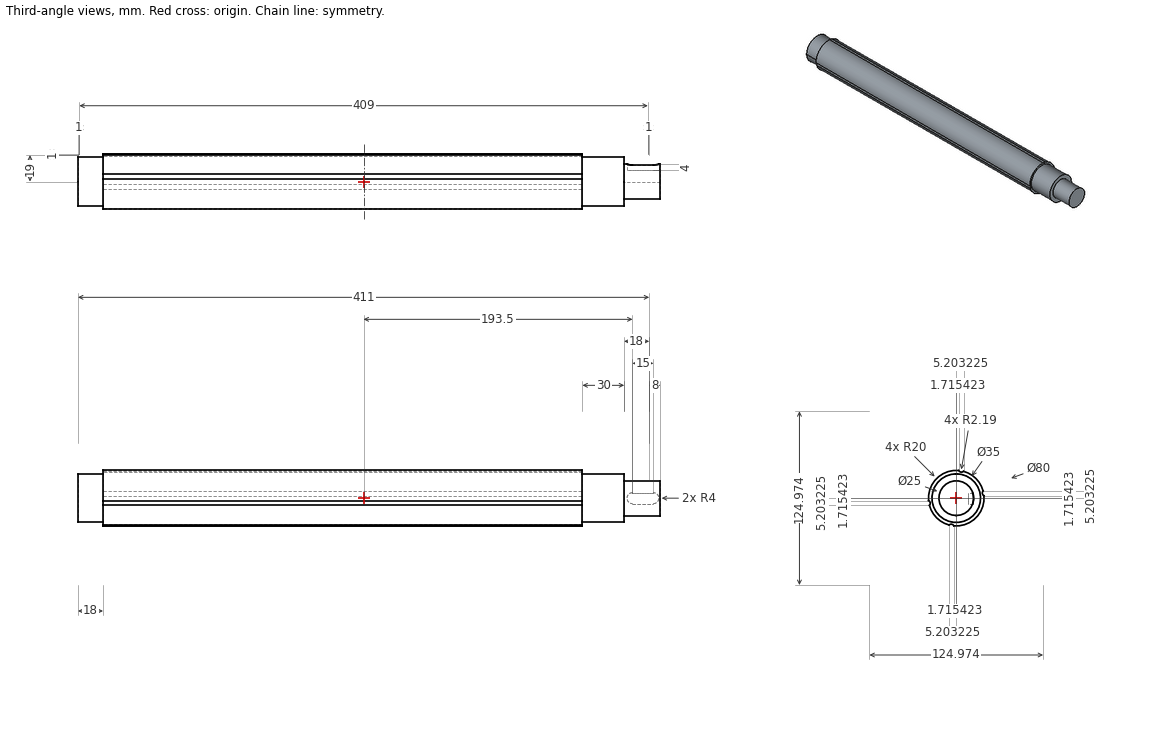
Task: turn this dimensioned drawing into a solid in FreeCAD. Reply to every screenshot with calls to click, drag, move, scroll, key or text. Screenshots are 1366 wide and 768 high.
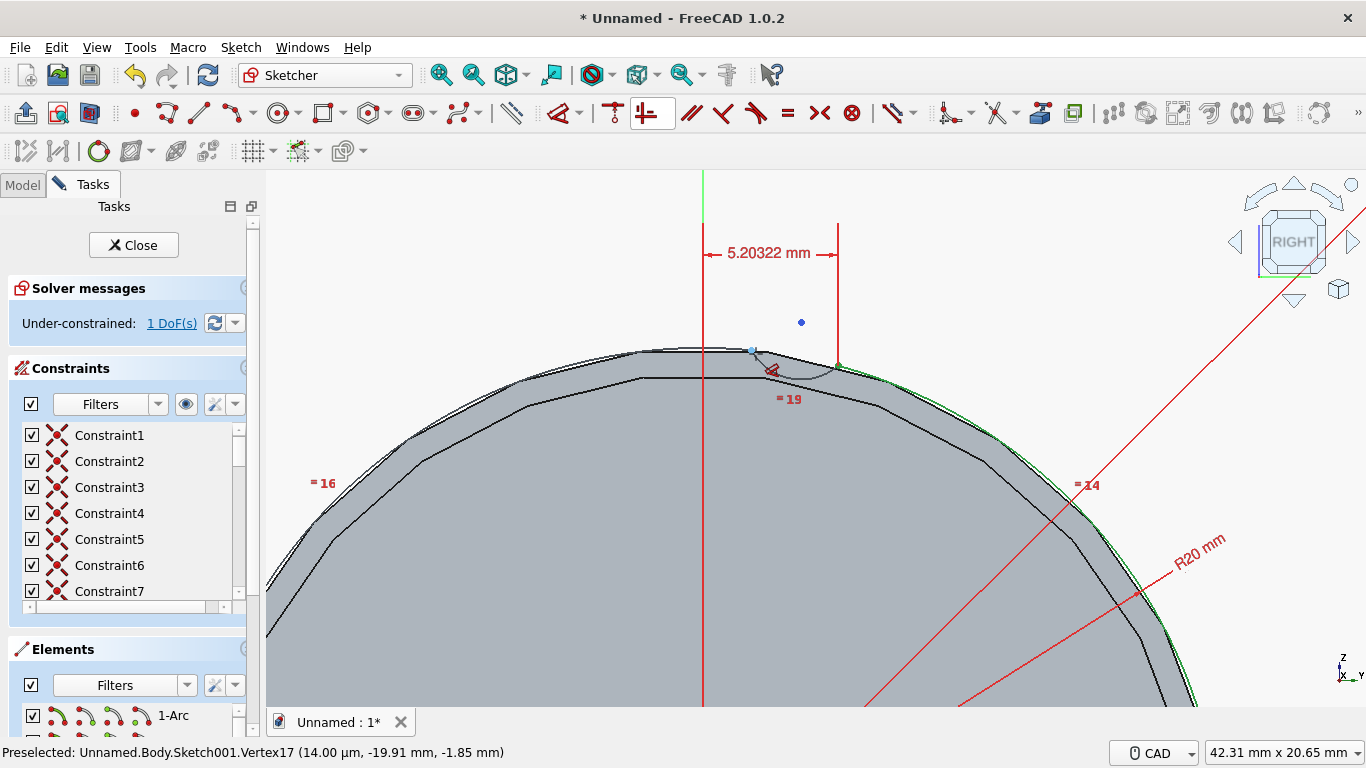
click(751, 350)
click(727, 316)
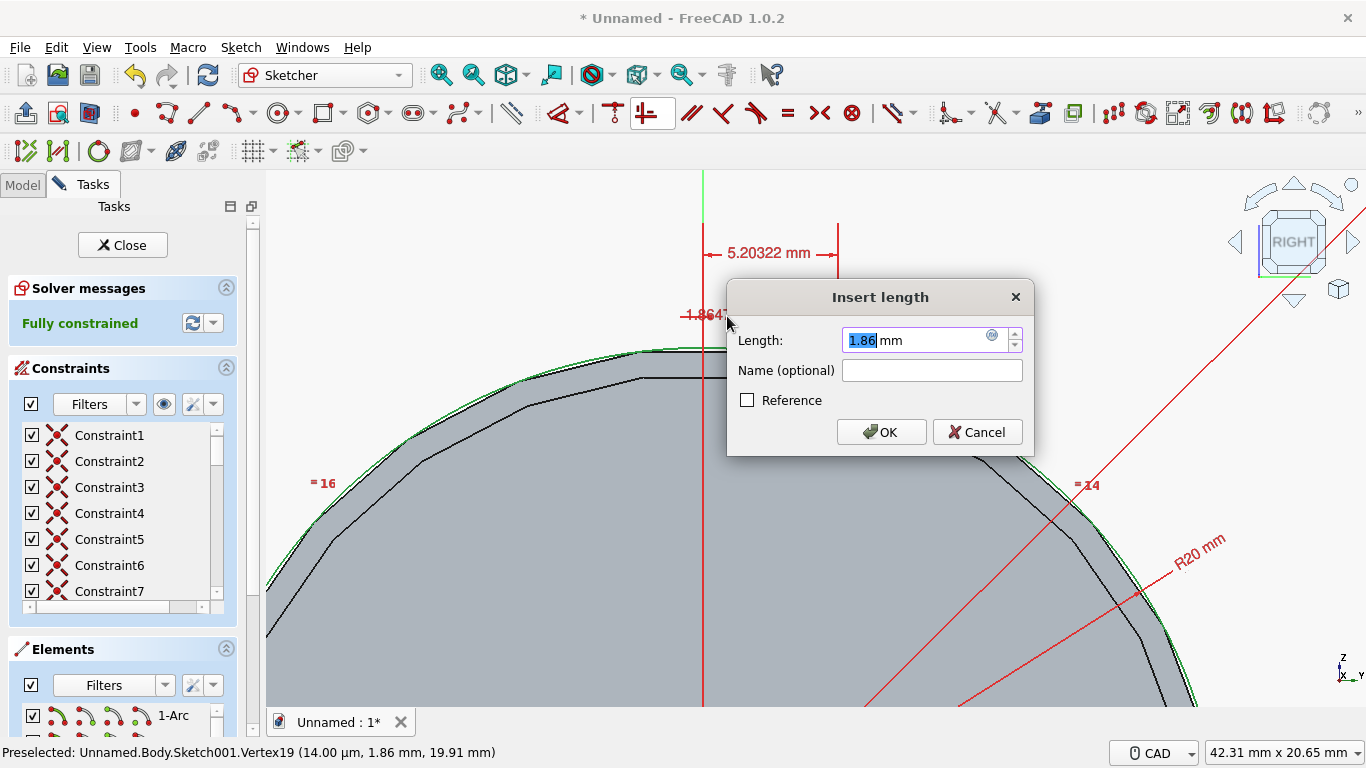
text(1.715423)
key(Return)
key(Escape)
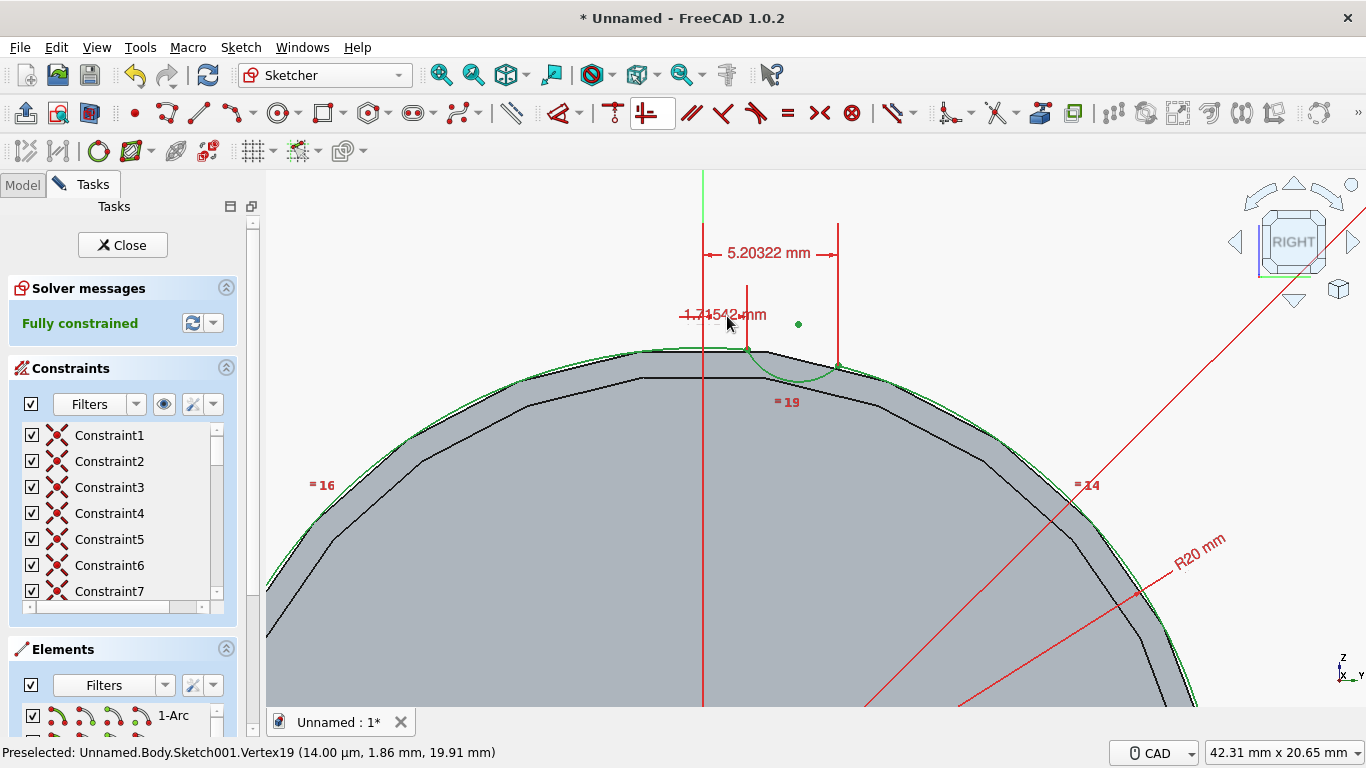
click(123, 245)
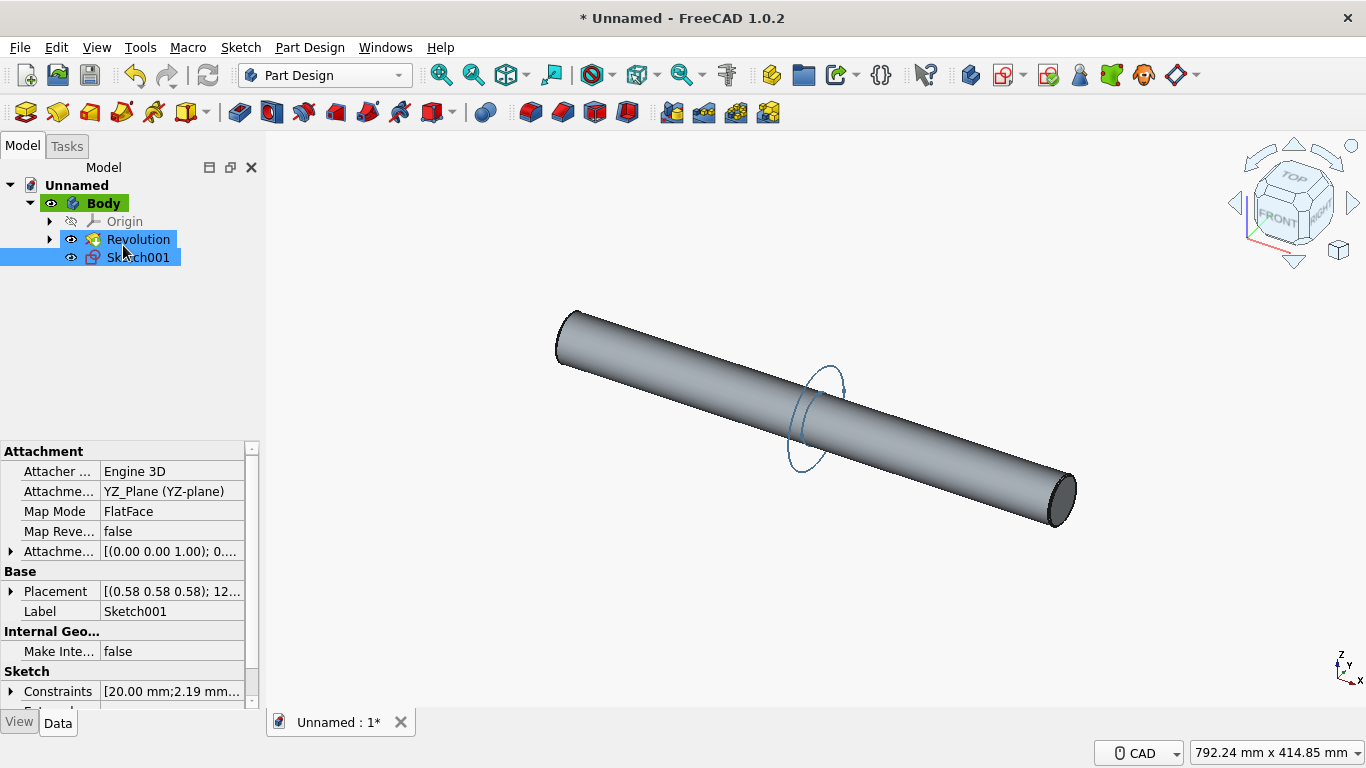
click(240, 112)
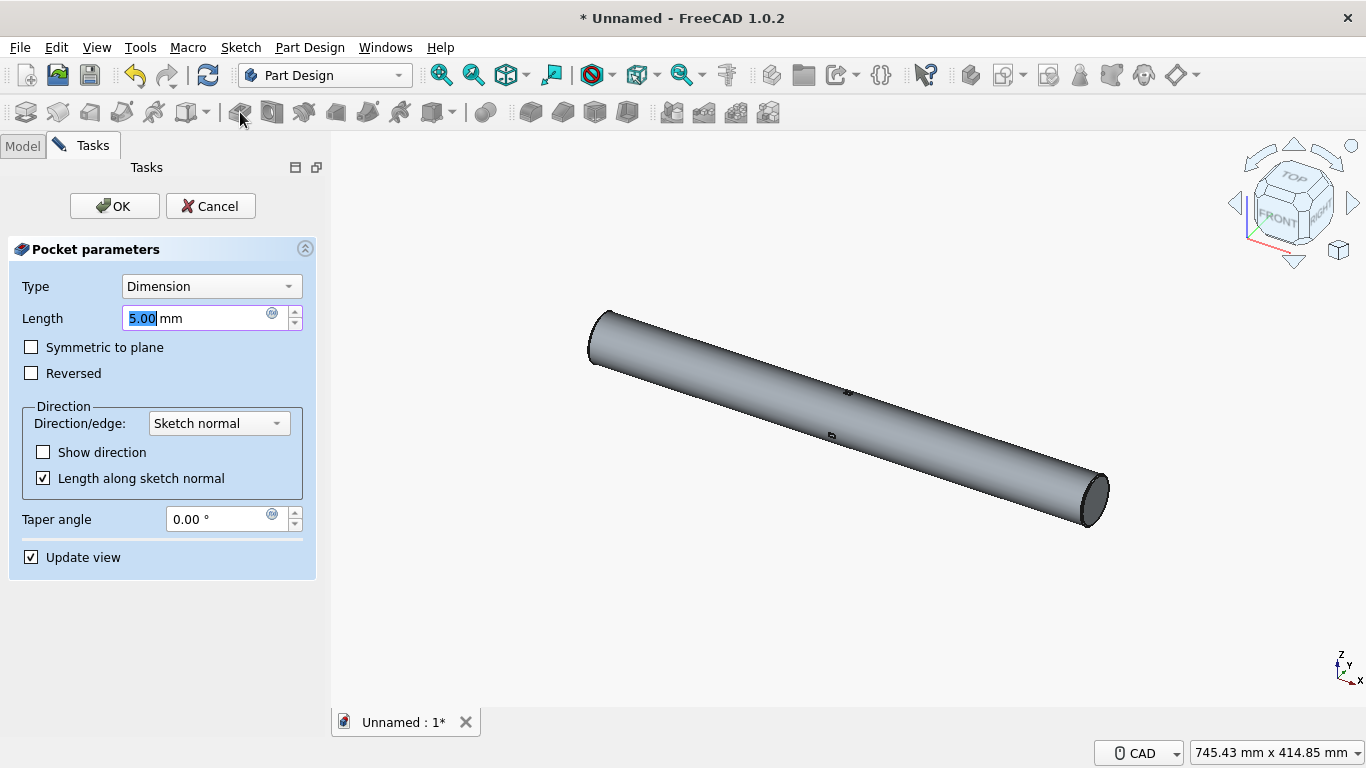
text(411)
key(Tab)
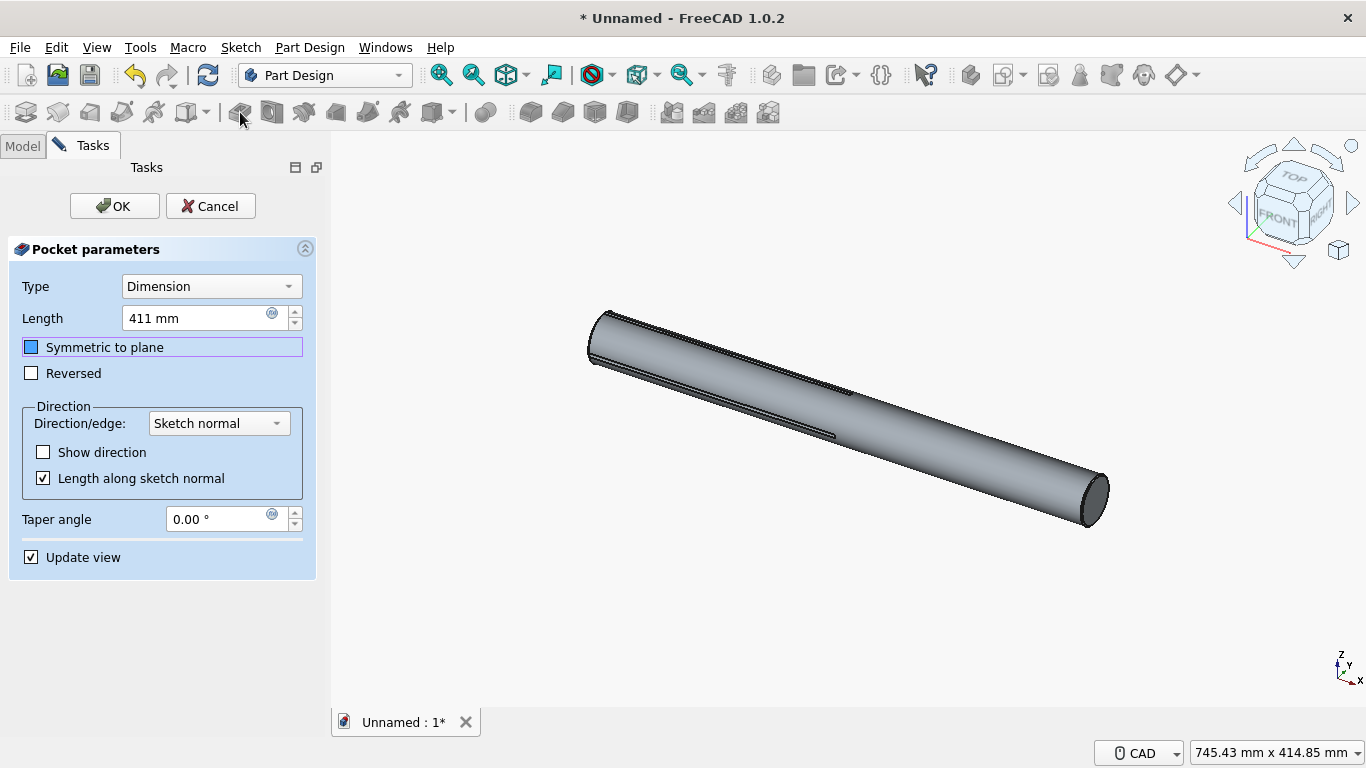
click(30, 347)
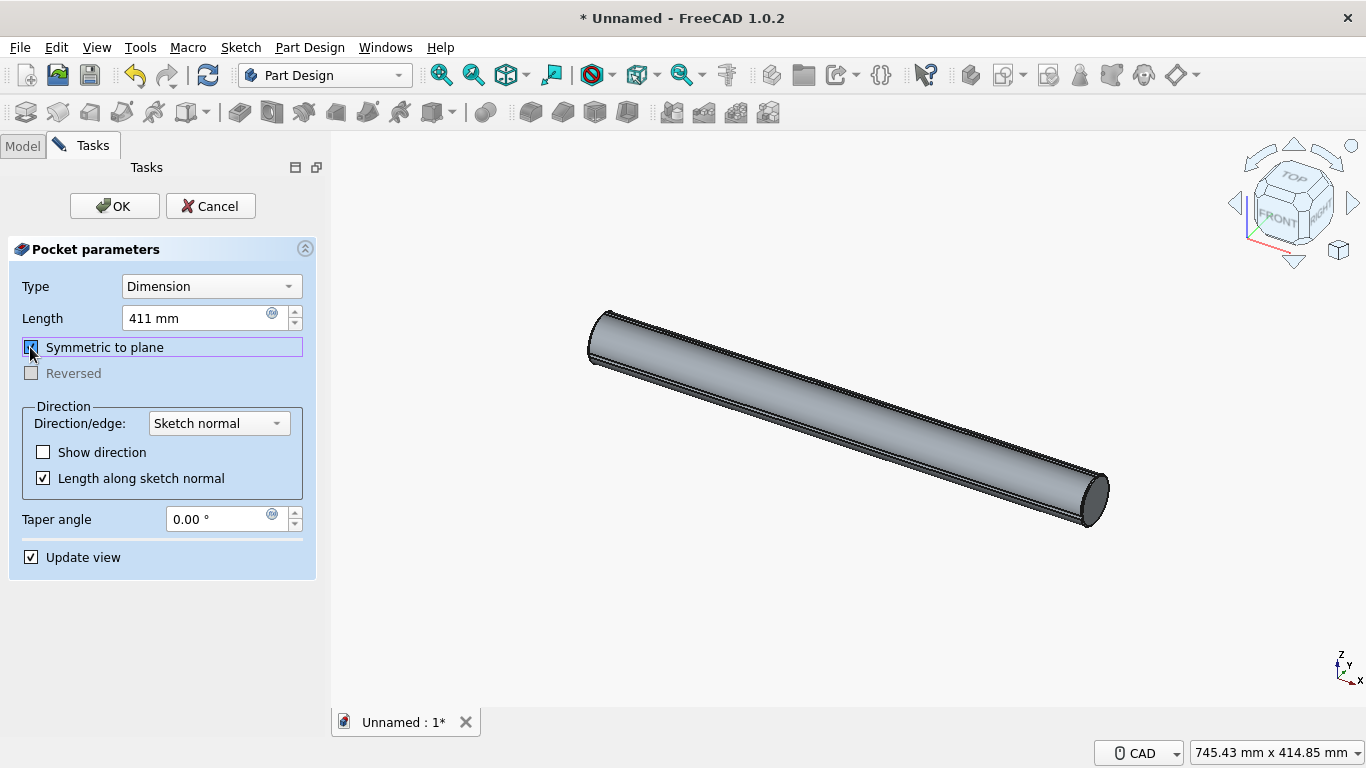
click(115, 206)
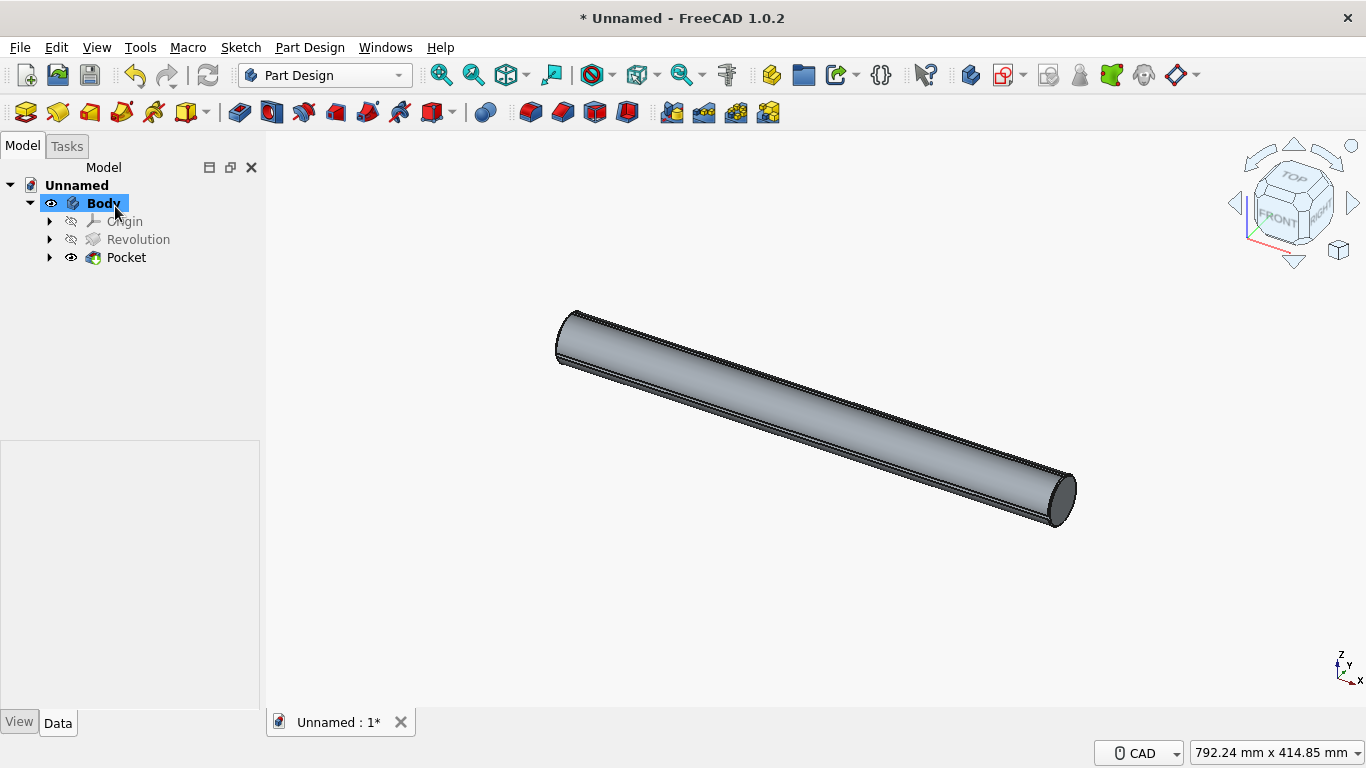
key(6)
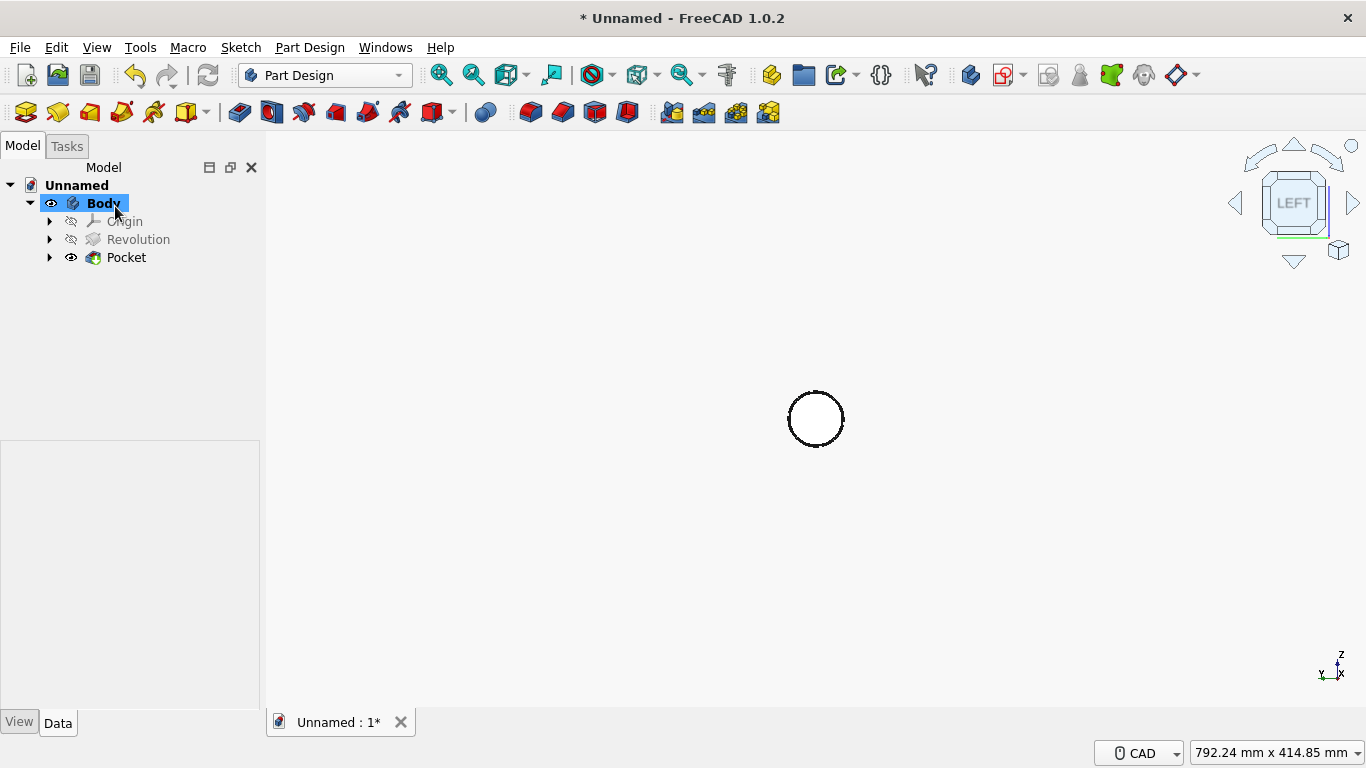
key(v)
key(f)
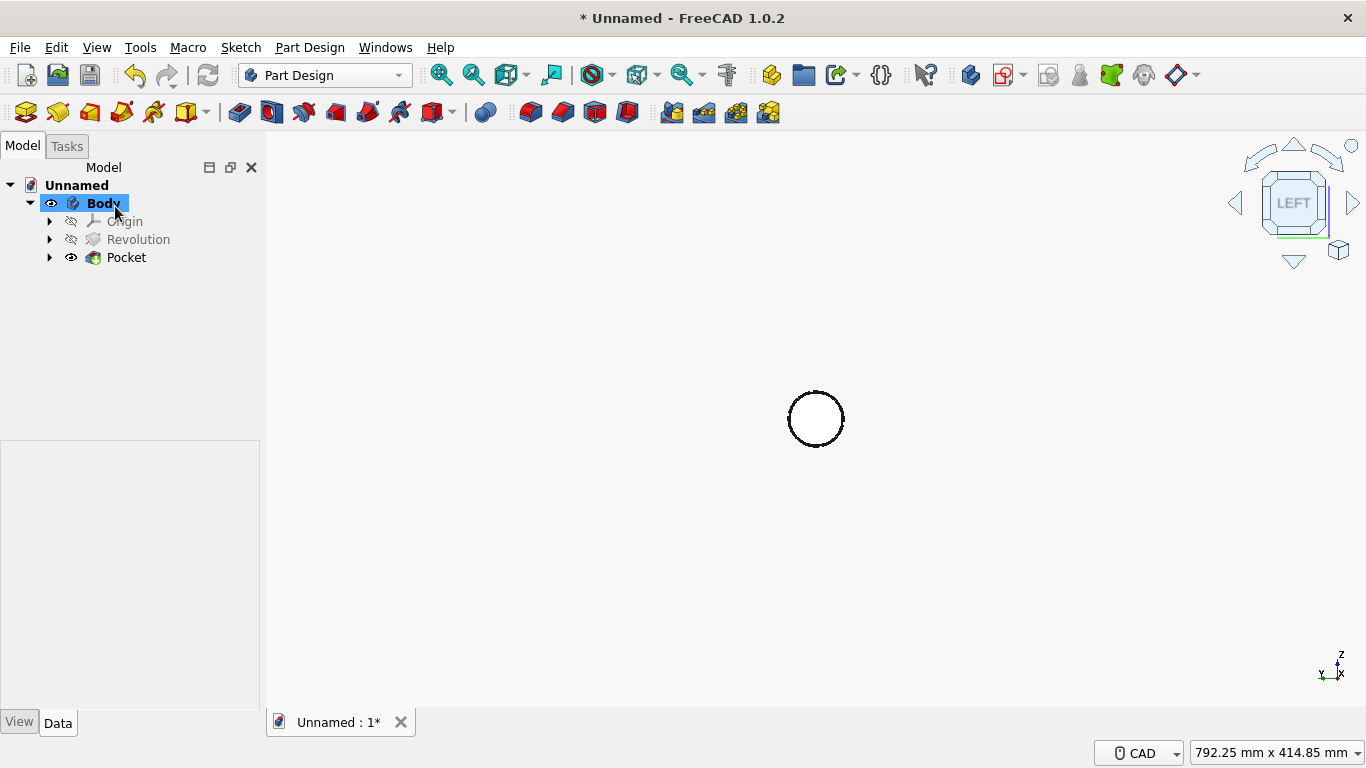
click(816, 418)